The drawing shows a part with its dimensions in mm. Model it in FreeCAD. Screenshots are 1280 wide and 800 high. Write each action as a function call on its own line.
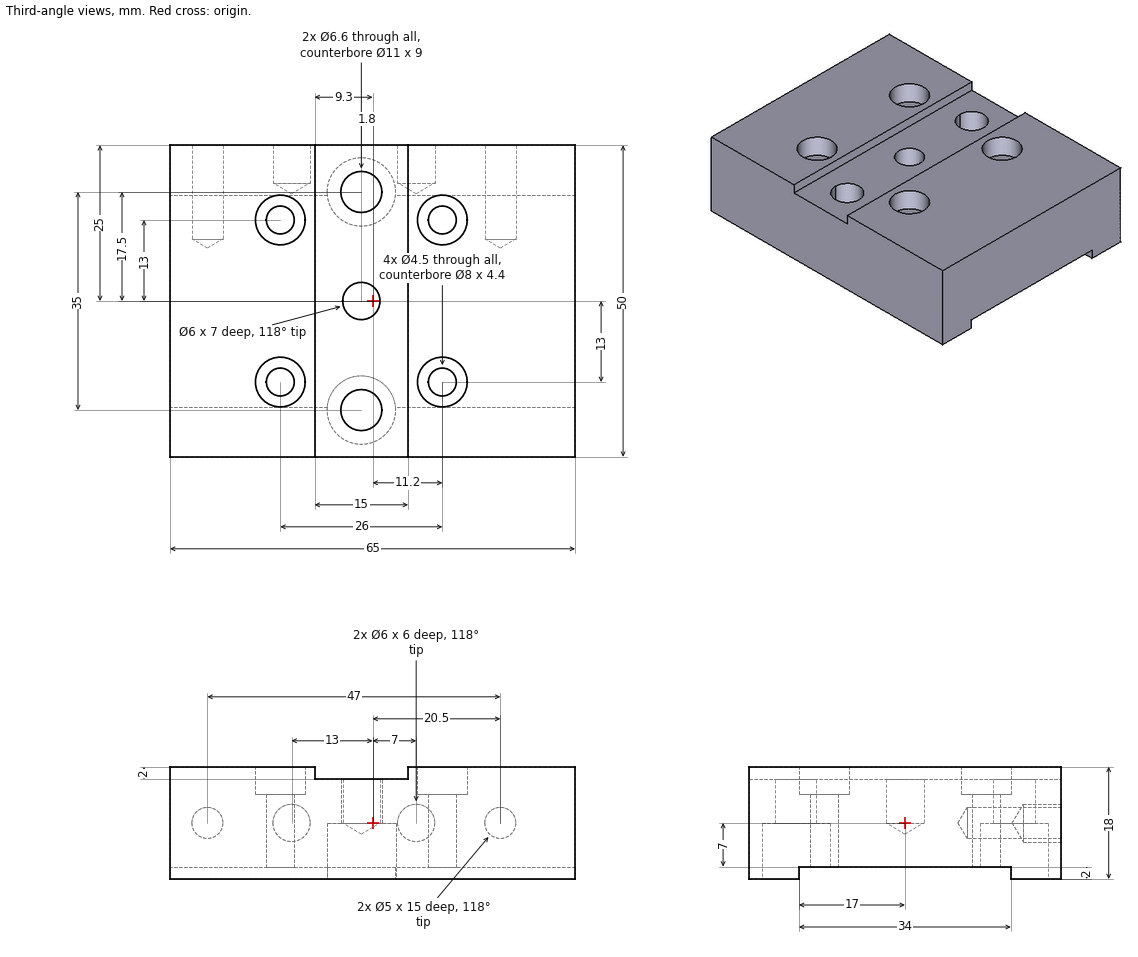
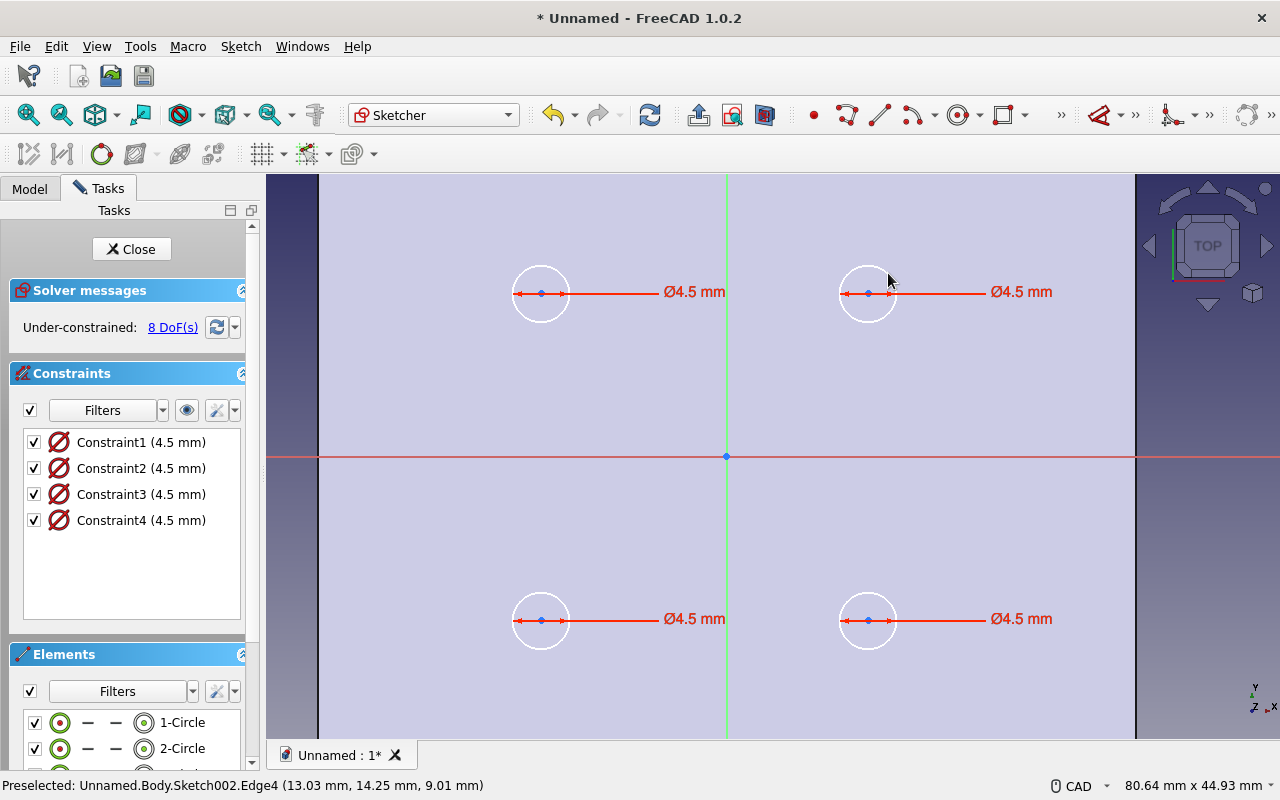
click(868, 621)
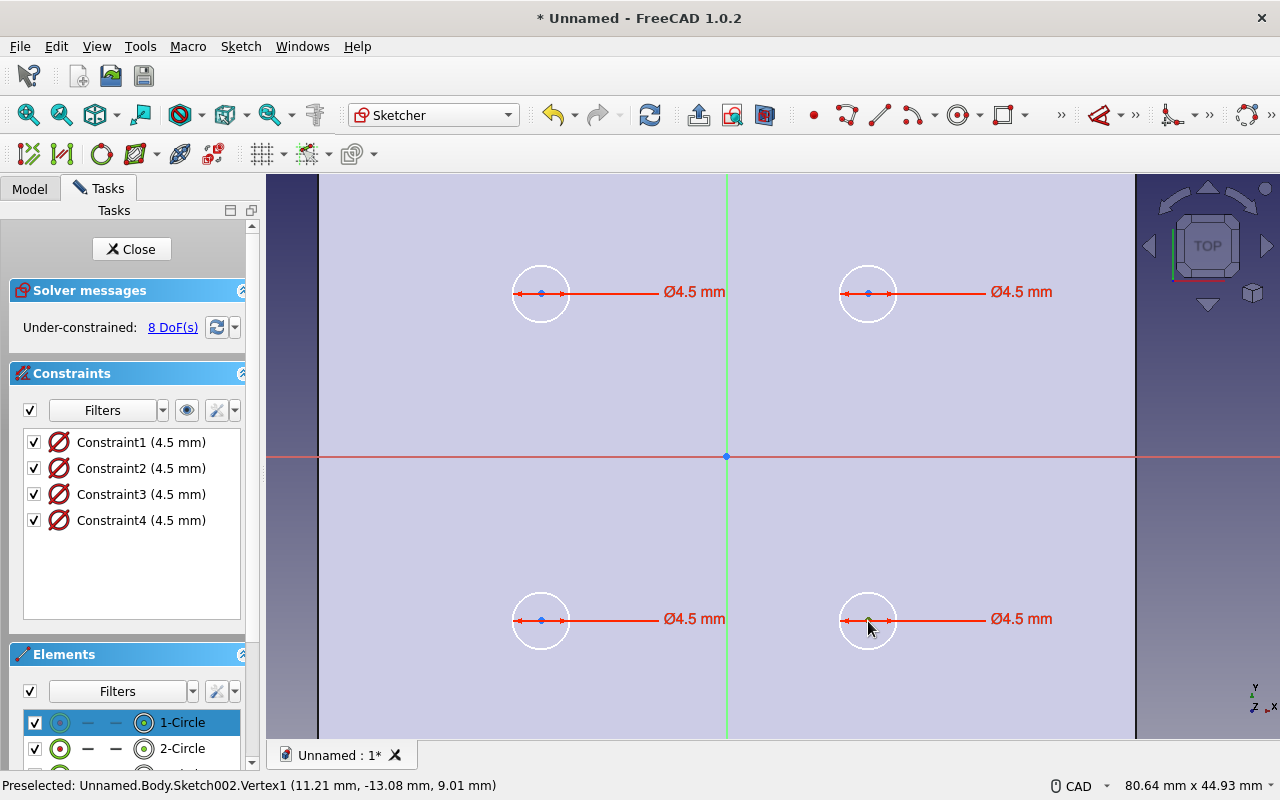
click(541, 621)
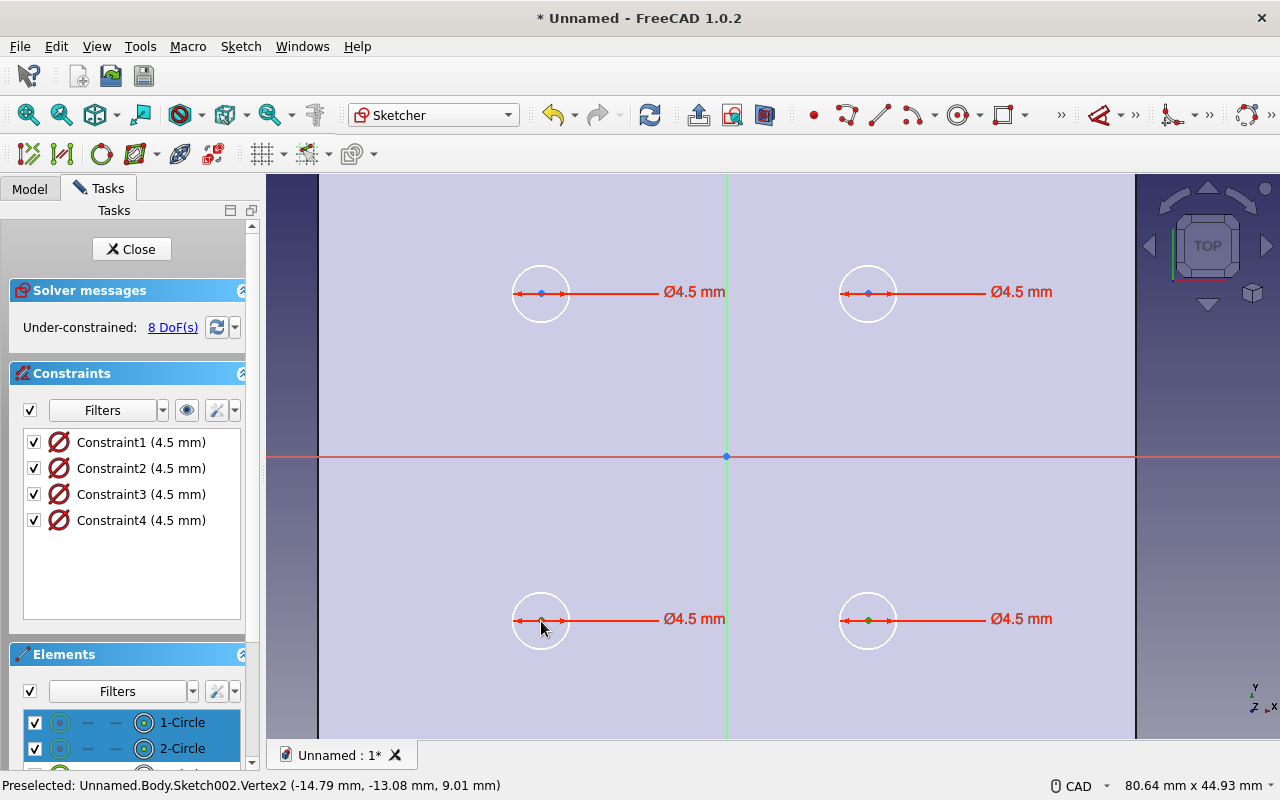
key(h)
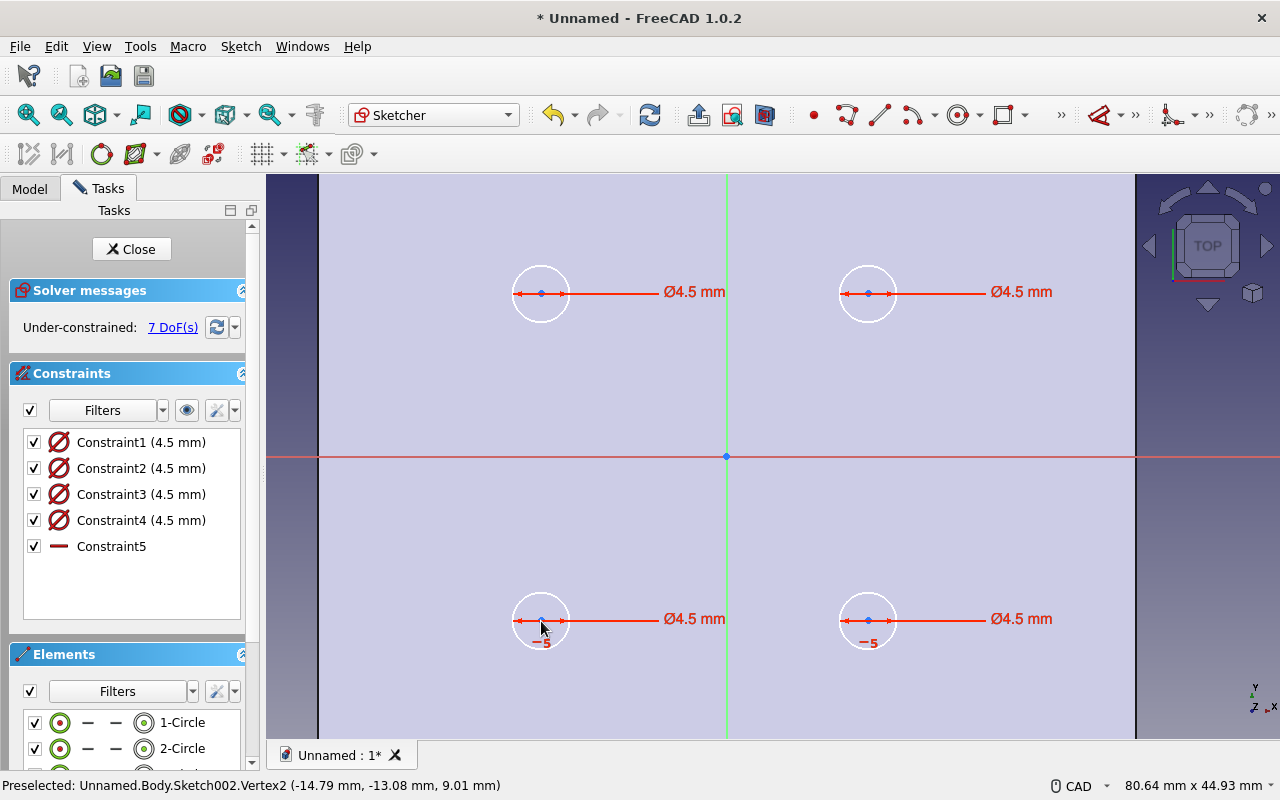
click(541, 621)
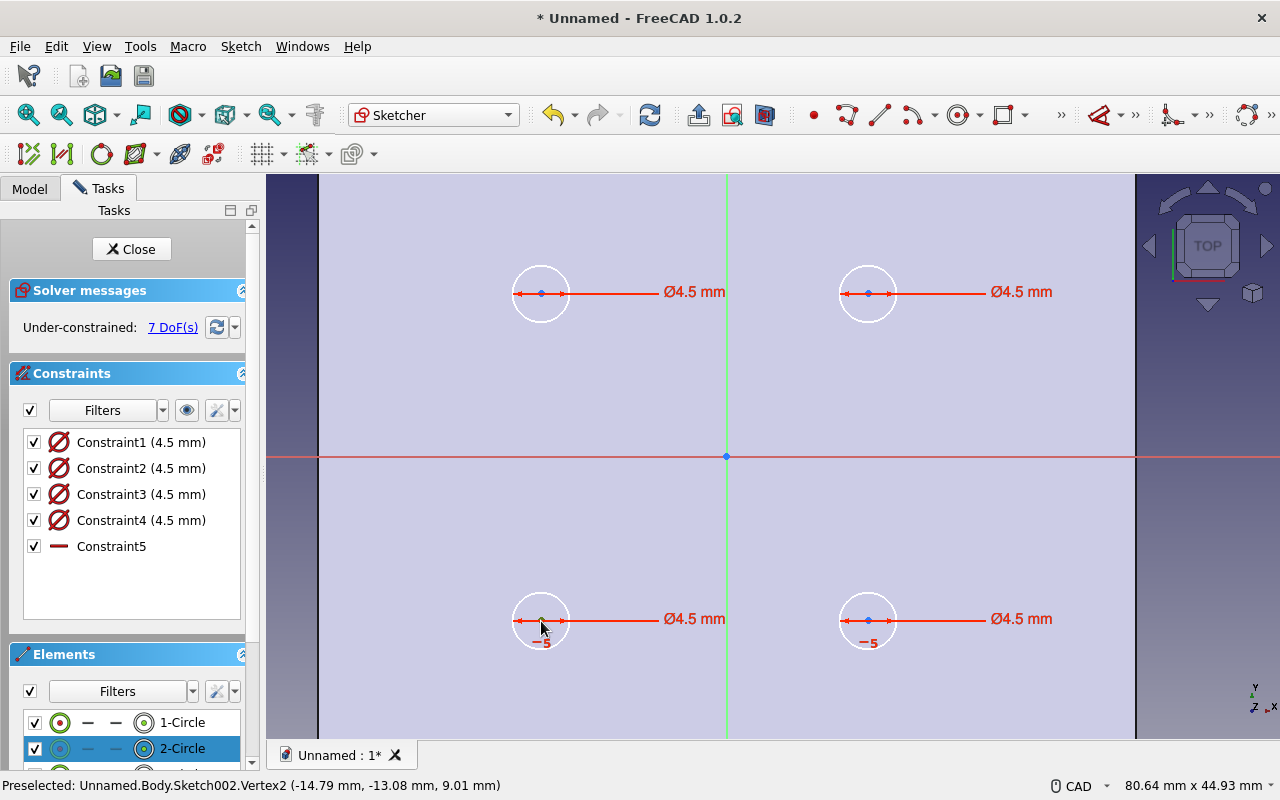
click(541, 294)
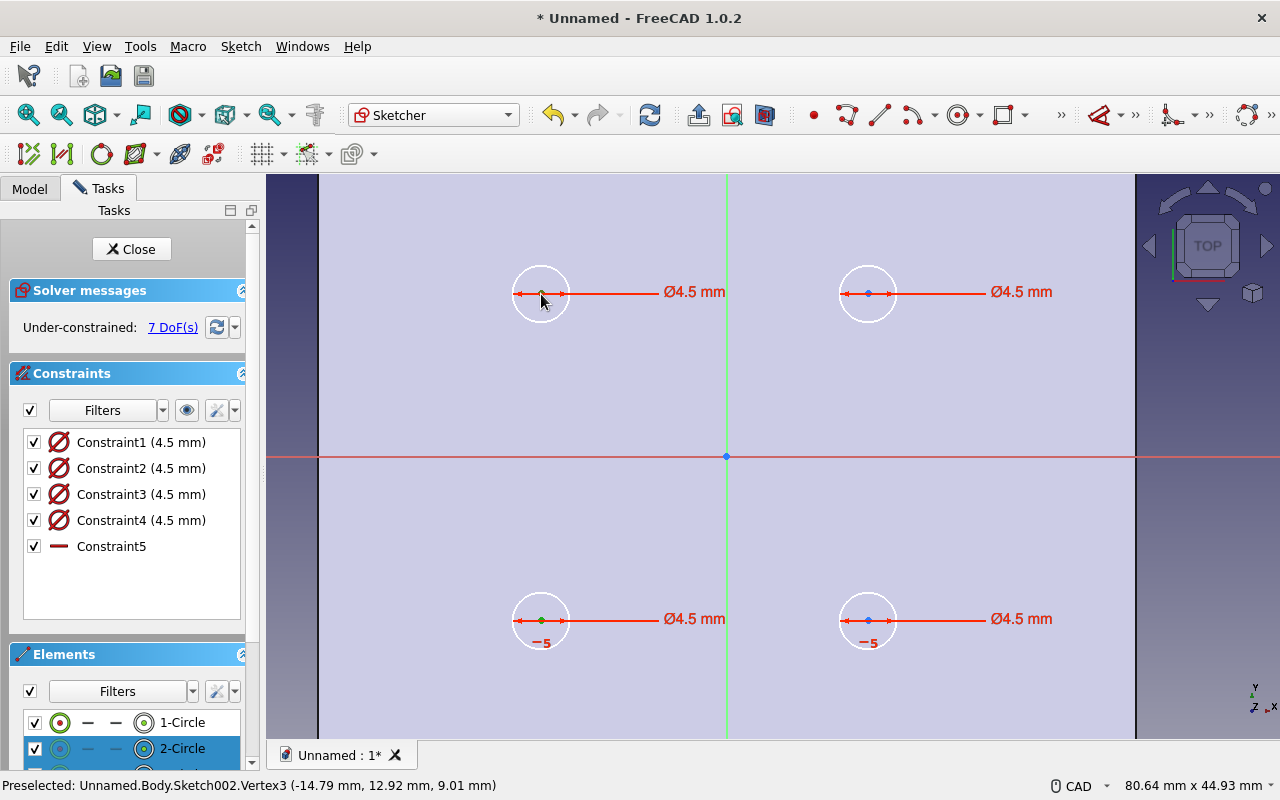
key(v)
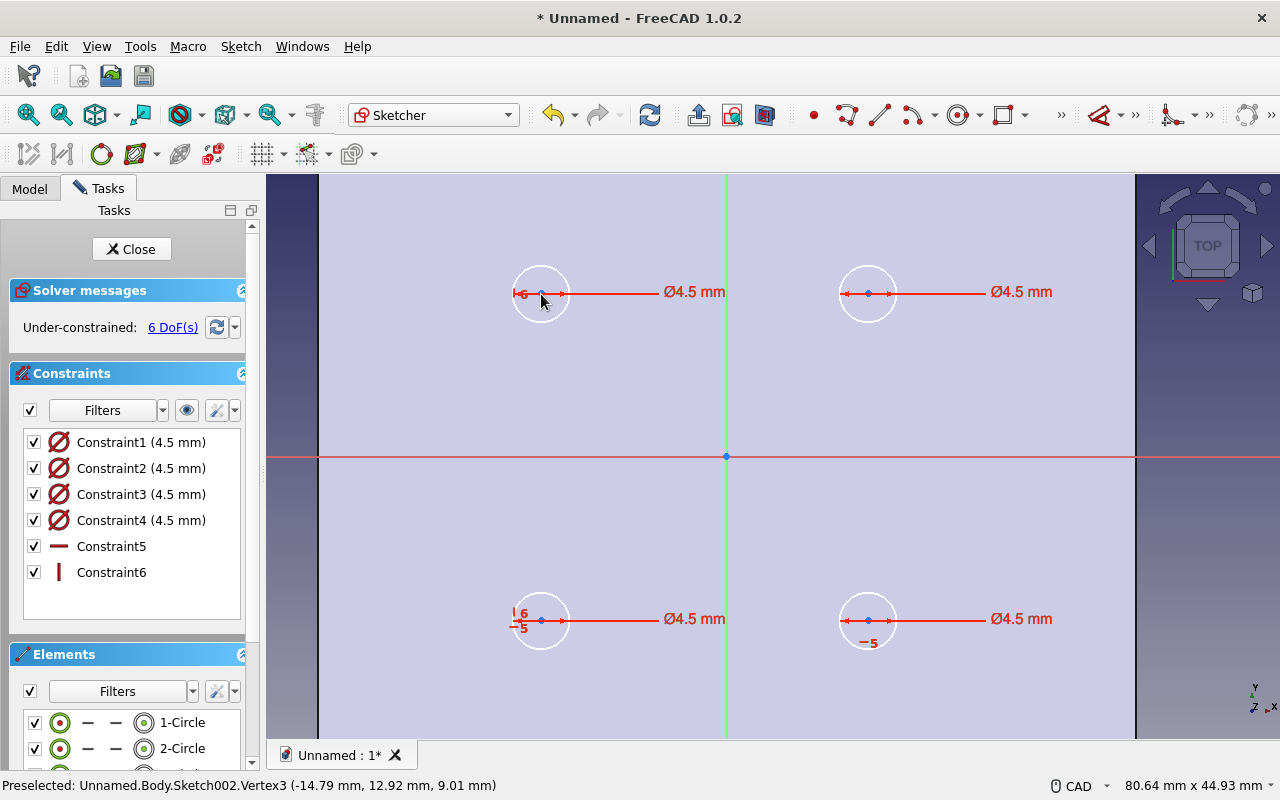
click(868, 621)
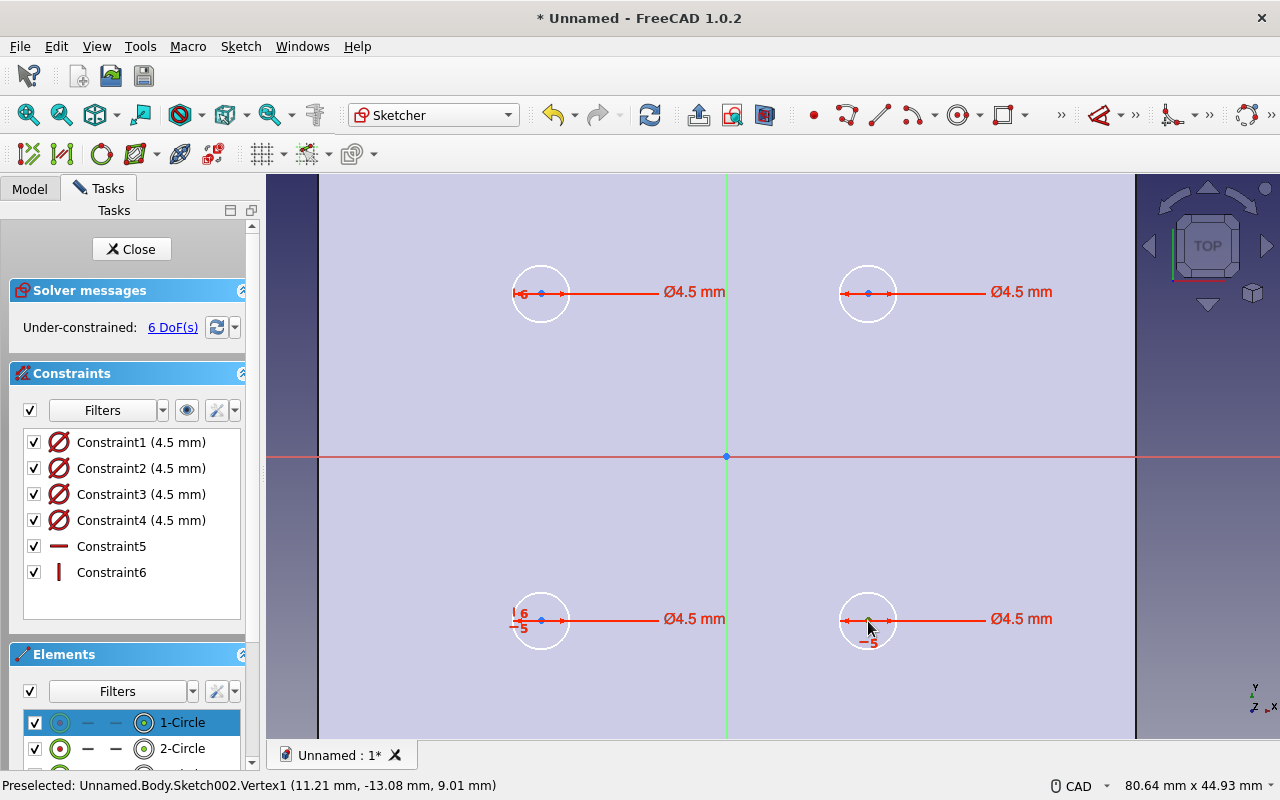
click(868, 294)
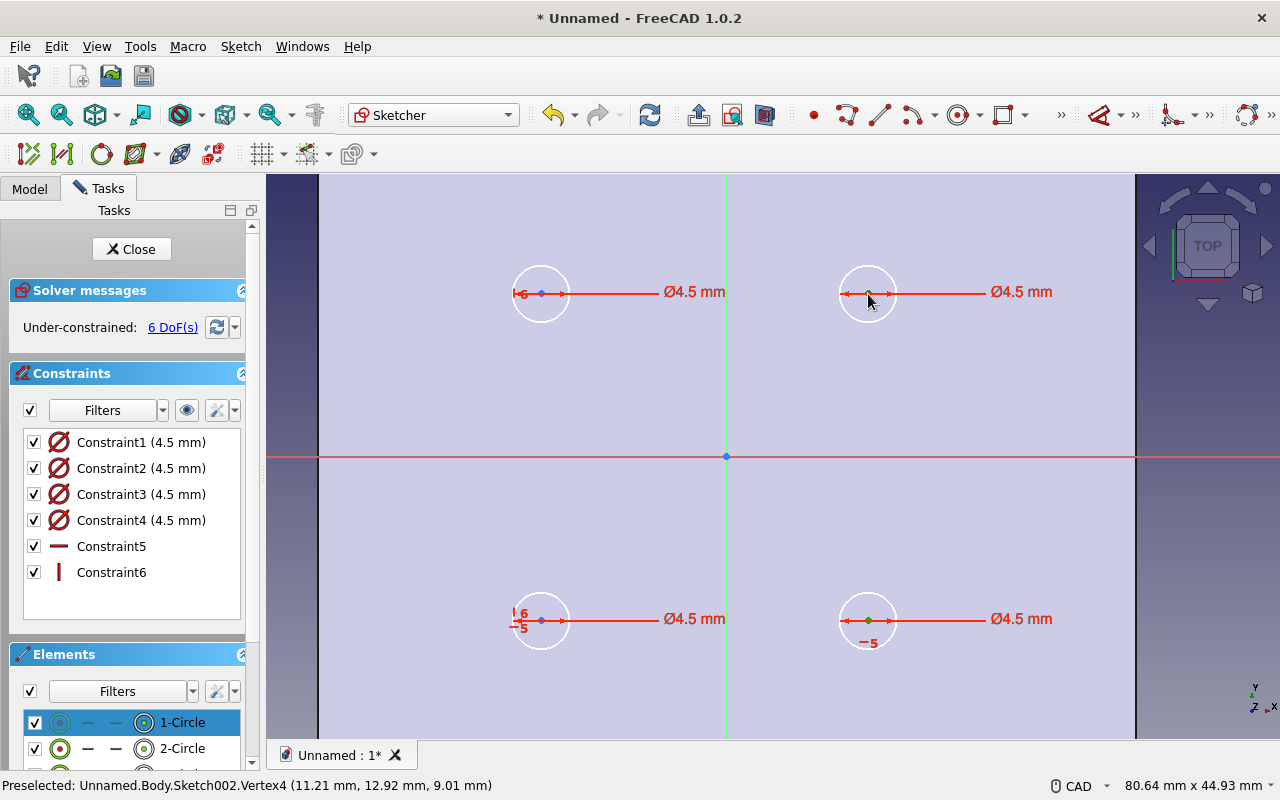
key(v)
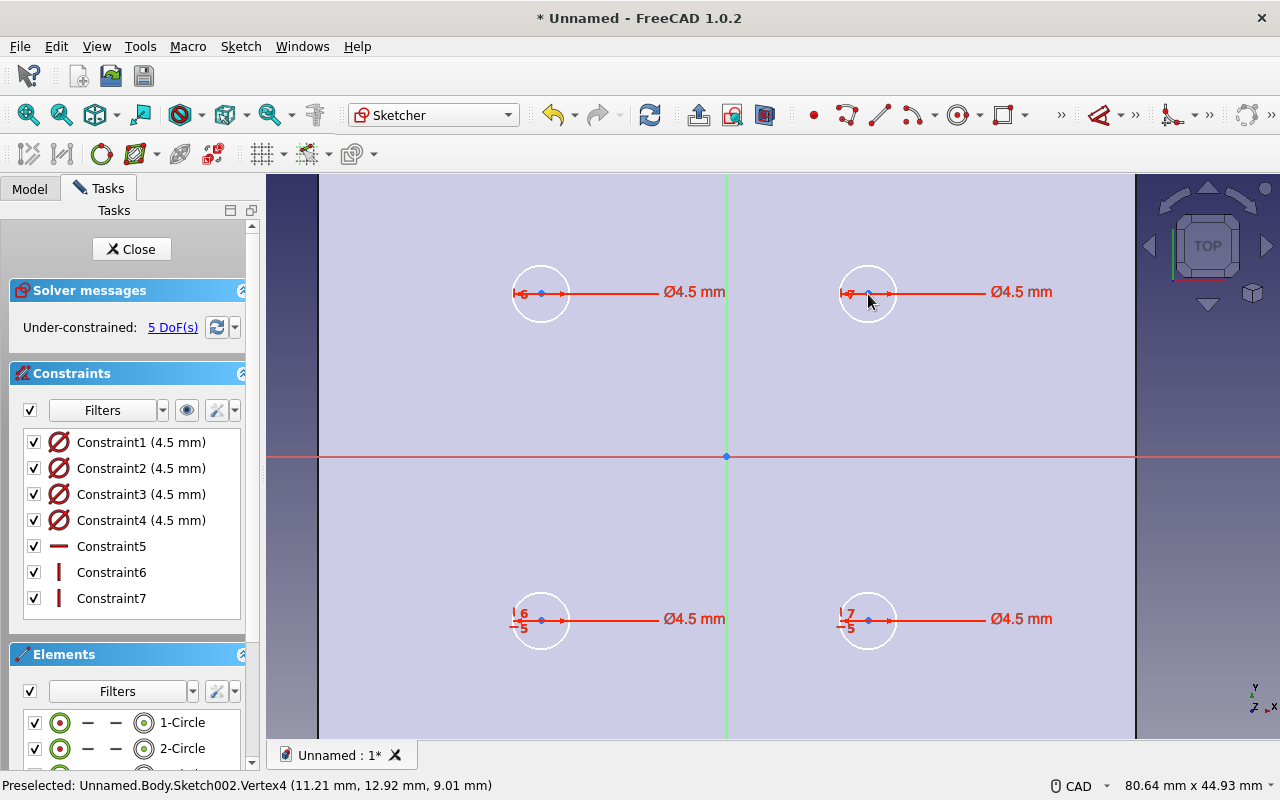
click(541, 294)